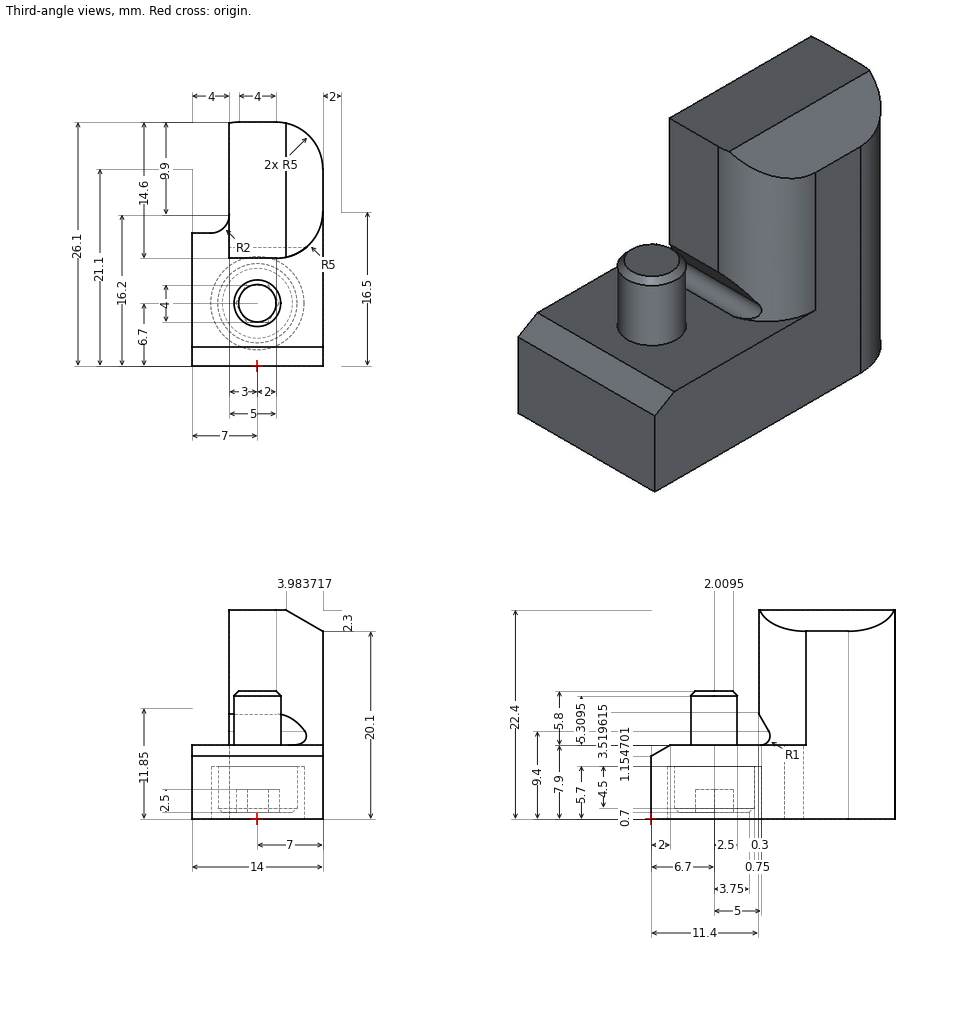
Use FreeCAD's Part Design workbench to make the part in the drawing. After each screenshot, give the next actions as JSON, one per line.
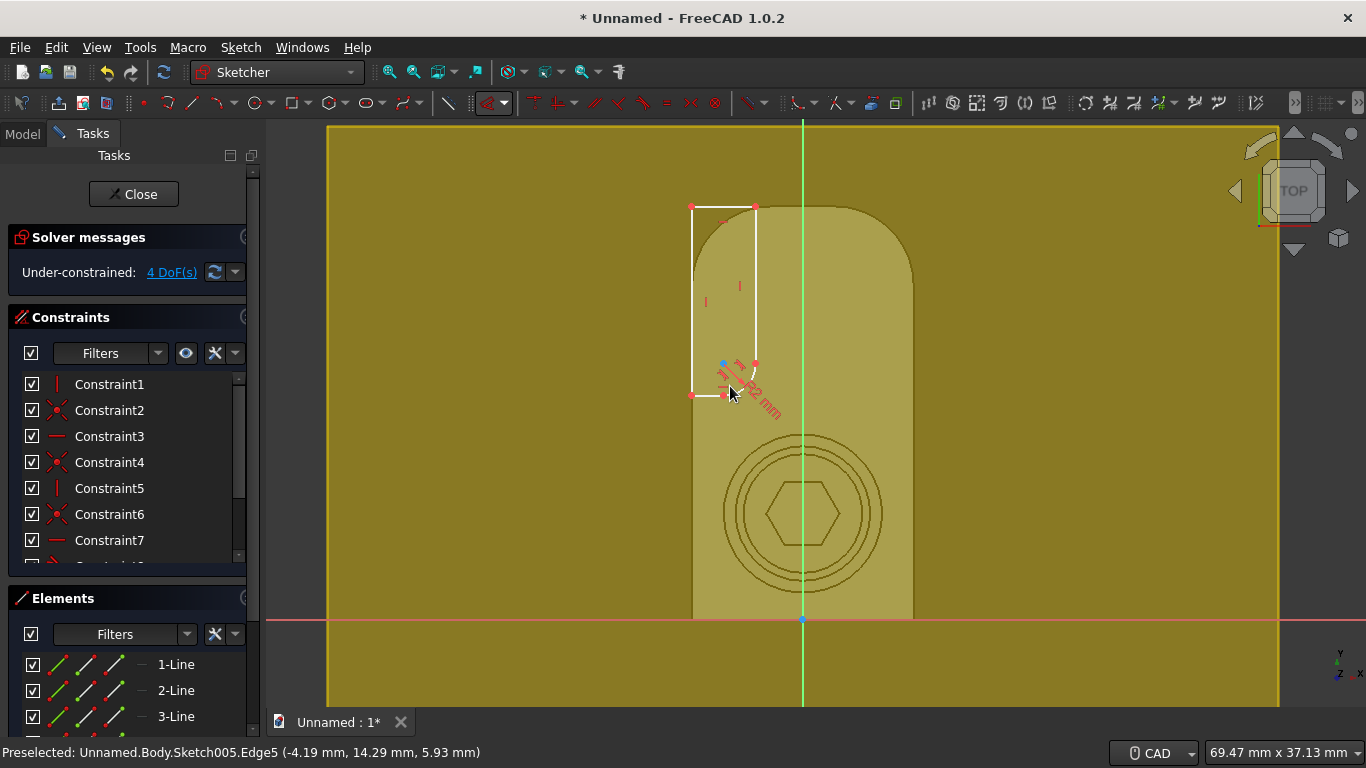
{"action": "left_click", "coordinate": [736, 207]}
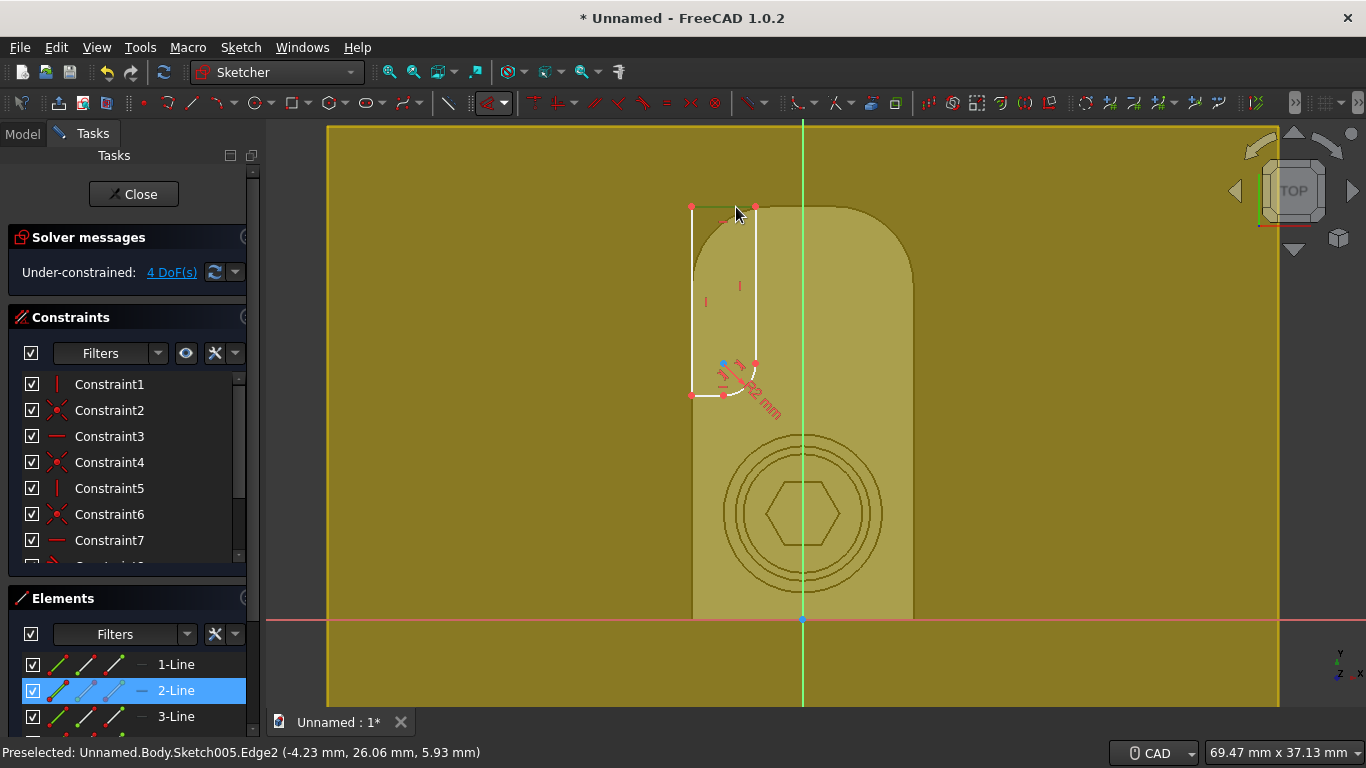
{"action": "key", "text": "l"}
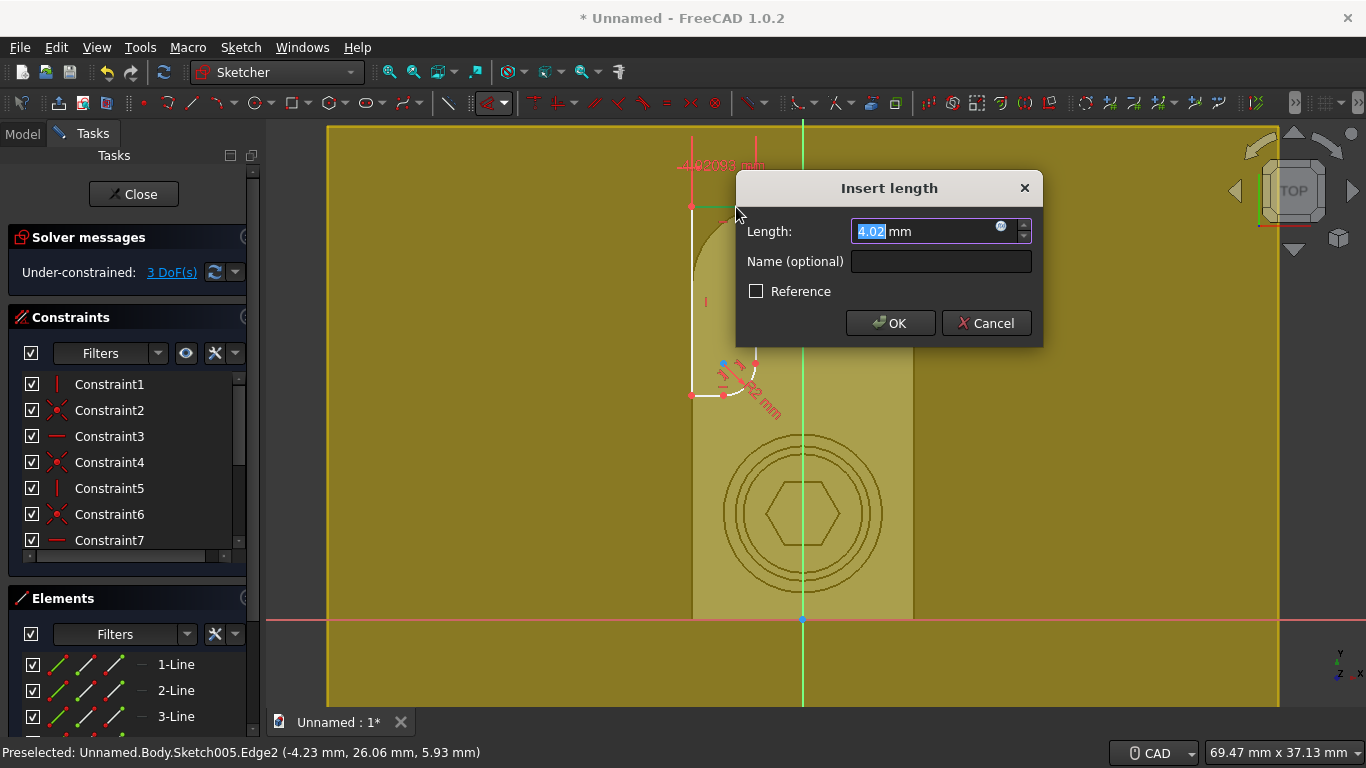
{"action": "type", "text": "4"}
{"action": "key", "text": "Return"}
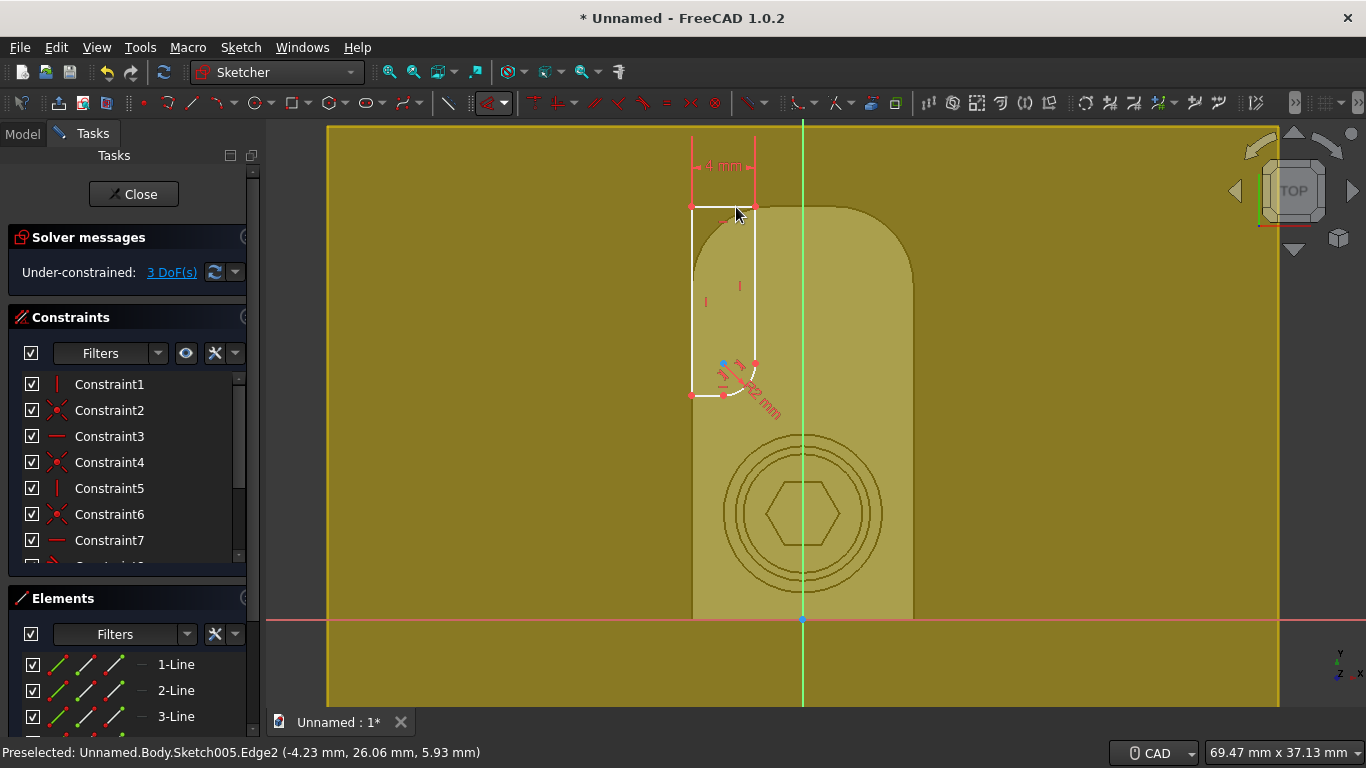
{"action": "left_click", "coordinate": [755, 364]}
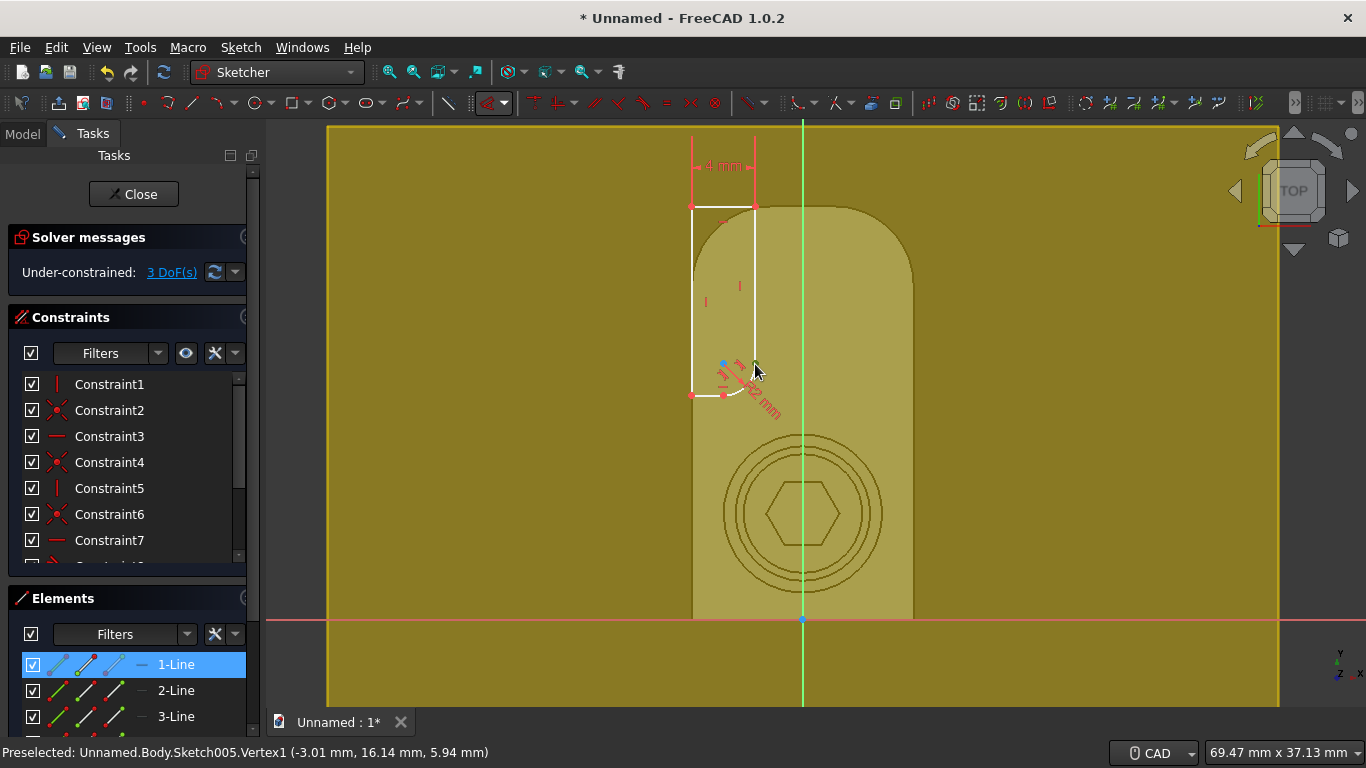
{"action": "key", "text": "l"}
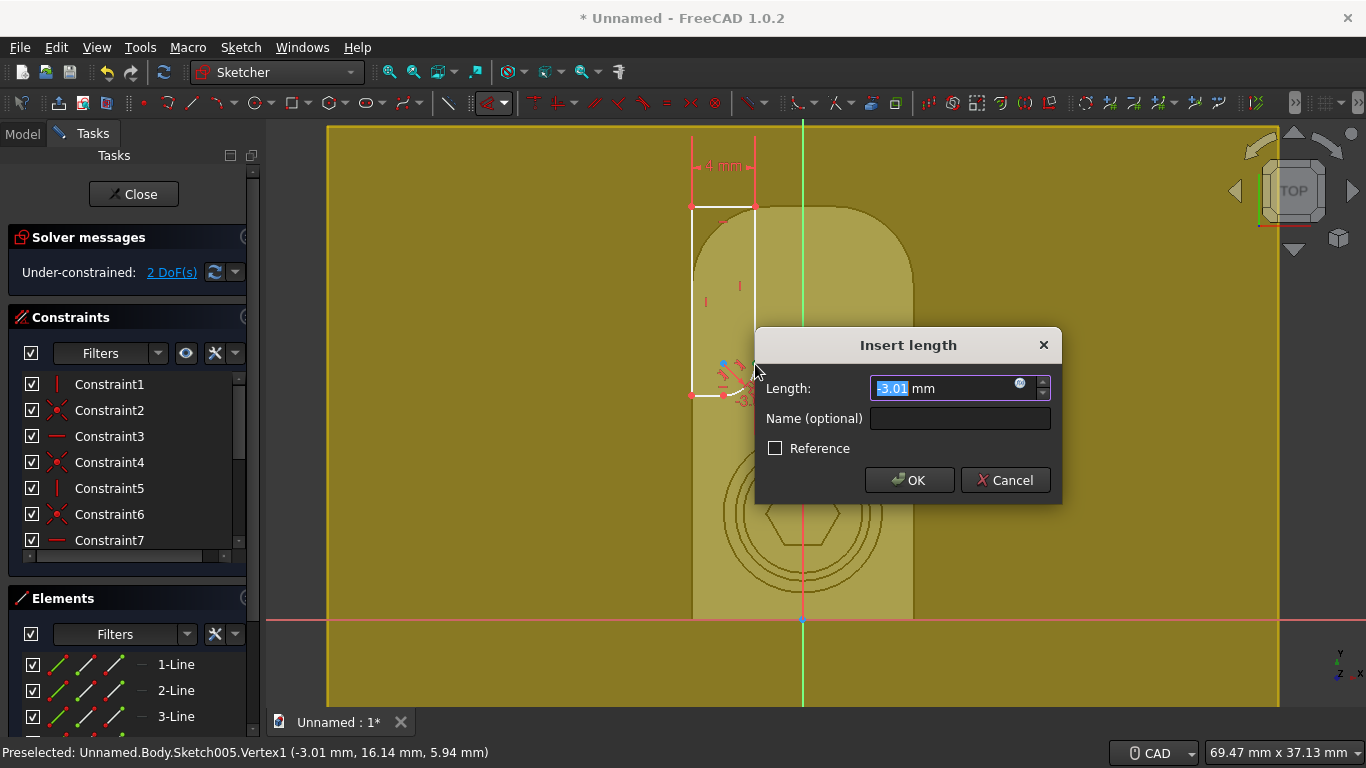
{"action": "type", "text": "-3"}
{"action": "key", "text": "Return"}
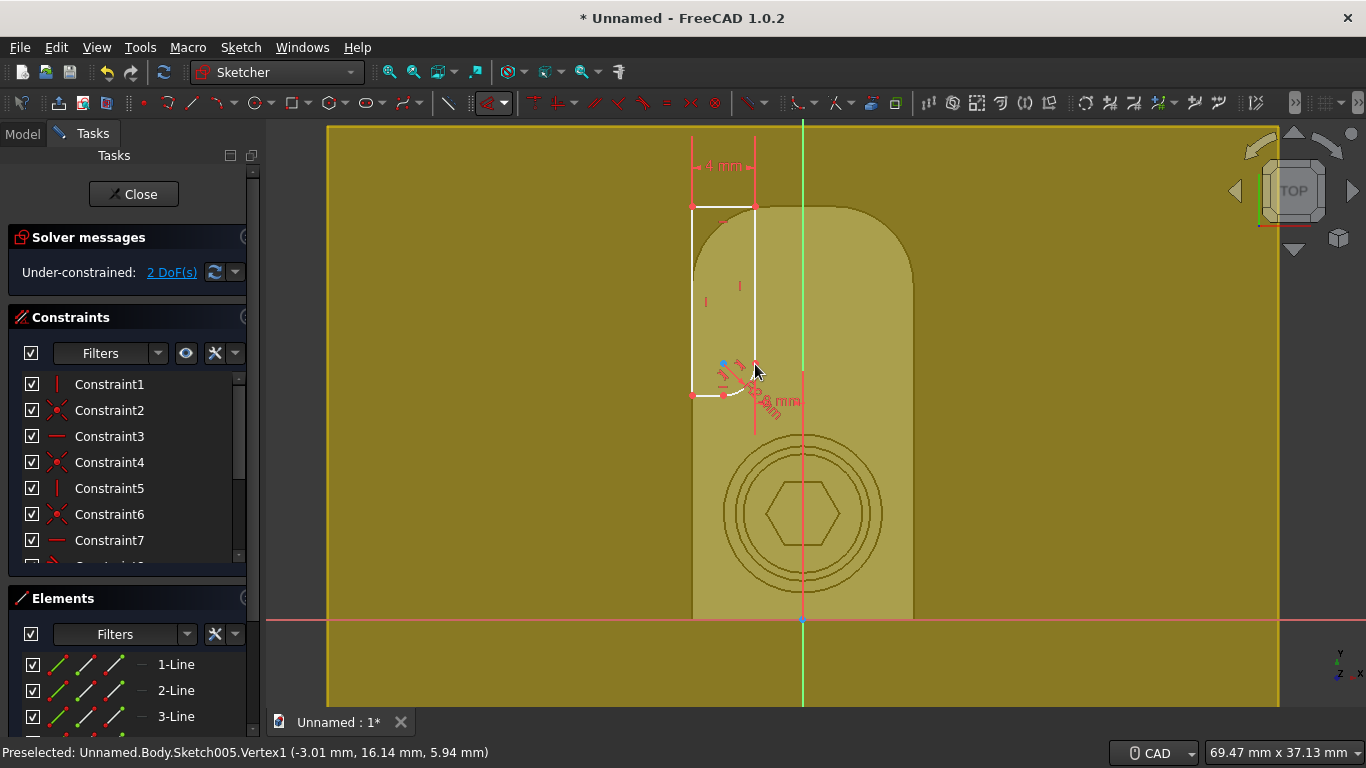
{"action": "left_click", "coordinate": [755, 317]}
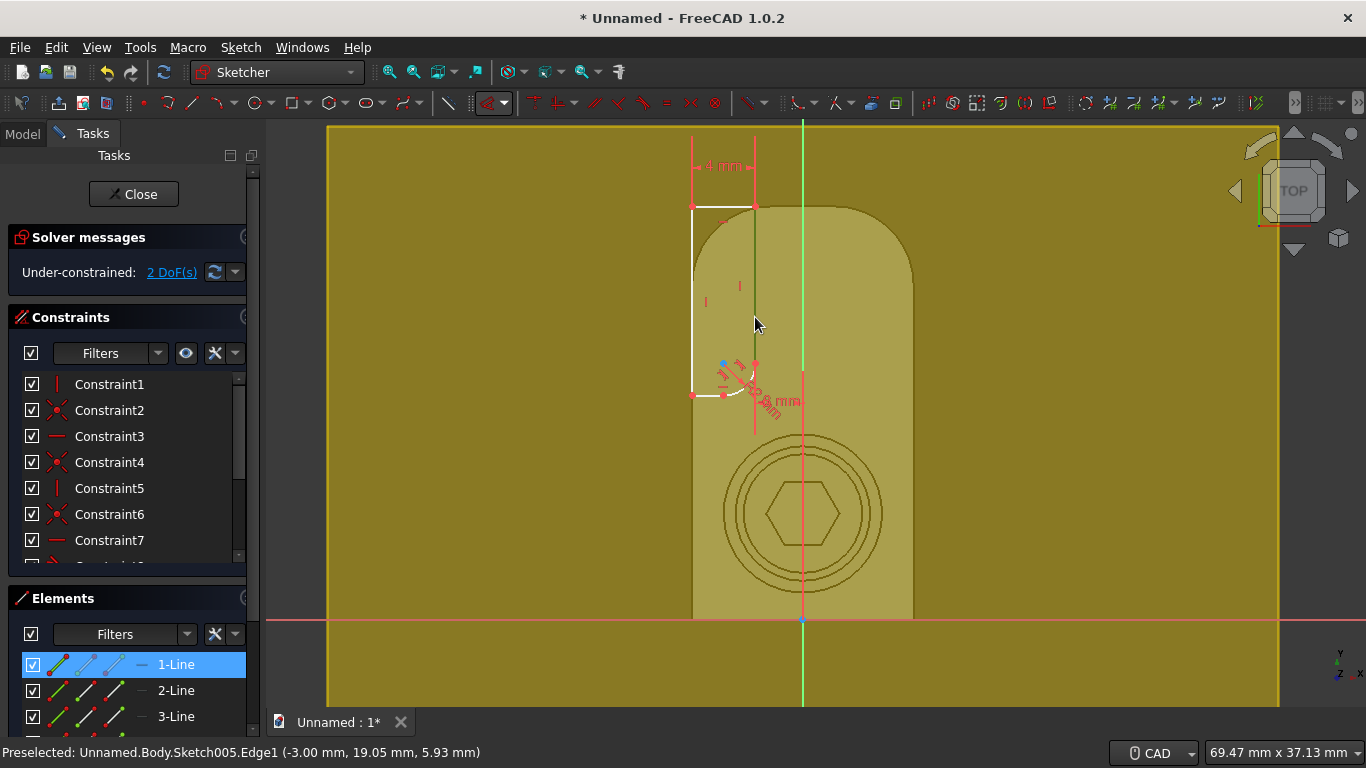
{"action": "left_click", "coordinate": [506, 104]}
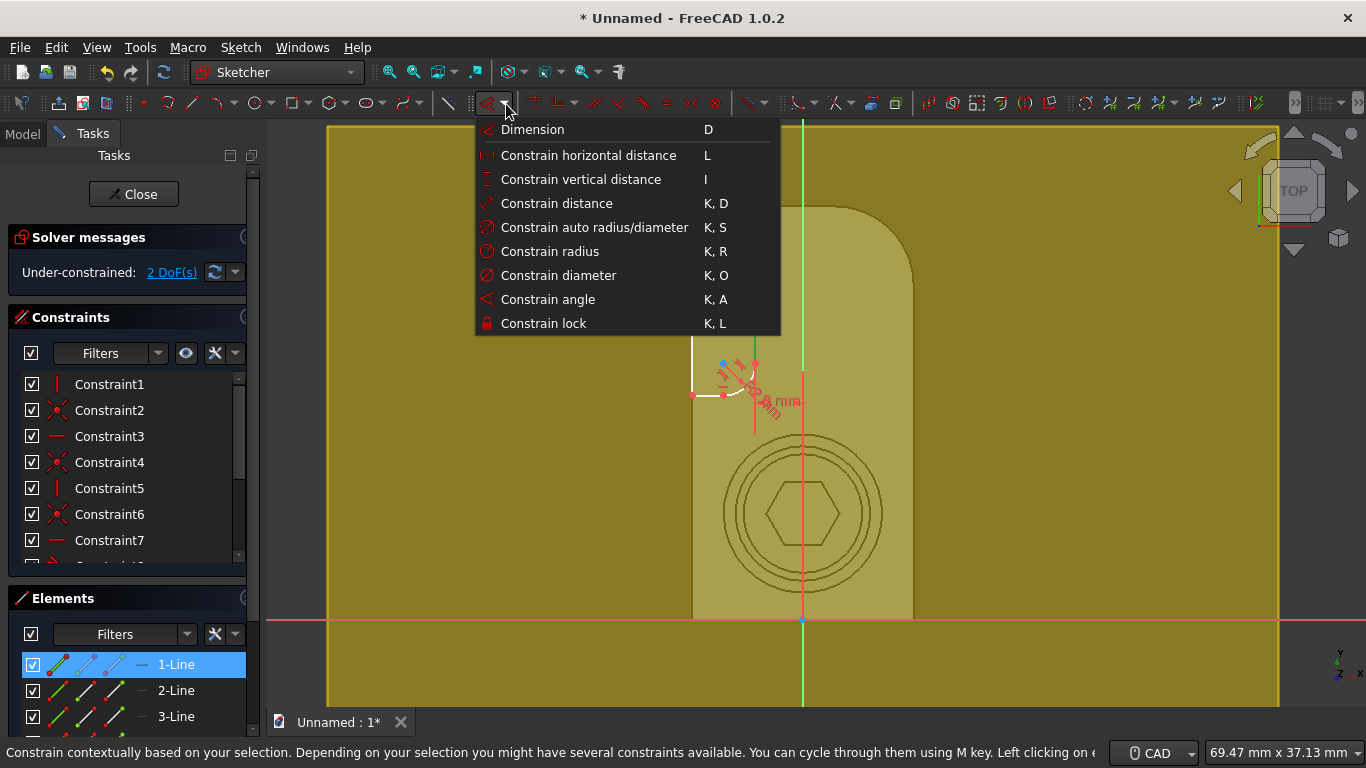
{"action": "left_click", "coordinate": [628, 179]}